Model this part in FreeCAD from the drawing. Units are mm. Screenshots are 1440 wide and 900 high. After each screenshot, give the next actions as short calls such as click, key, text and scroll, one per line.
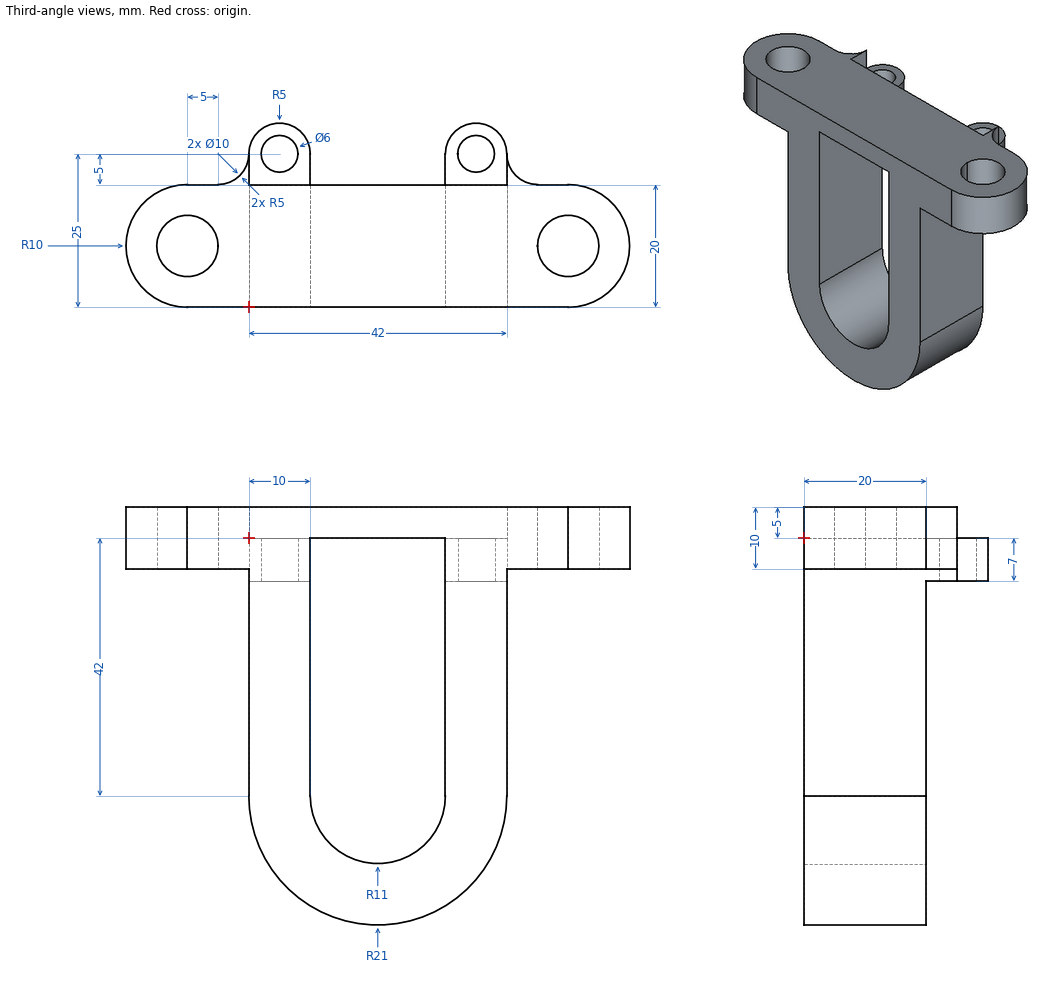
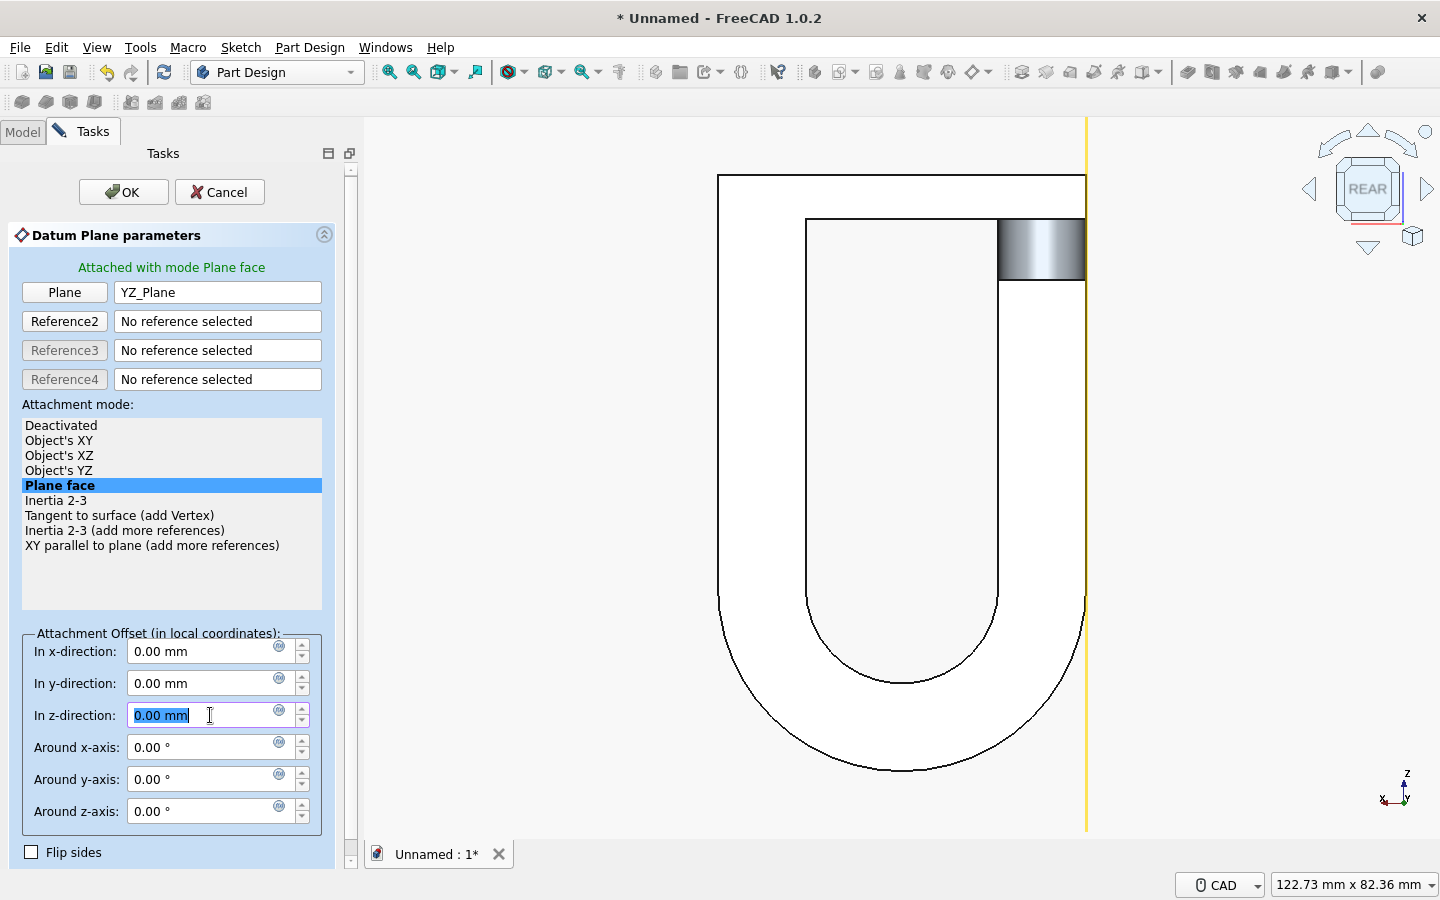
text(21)
key(Tab)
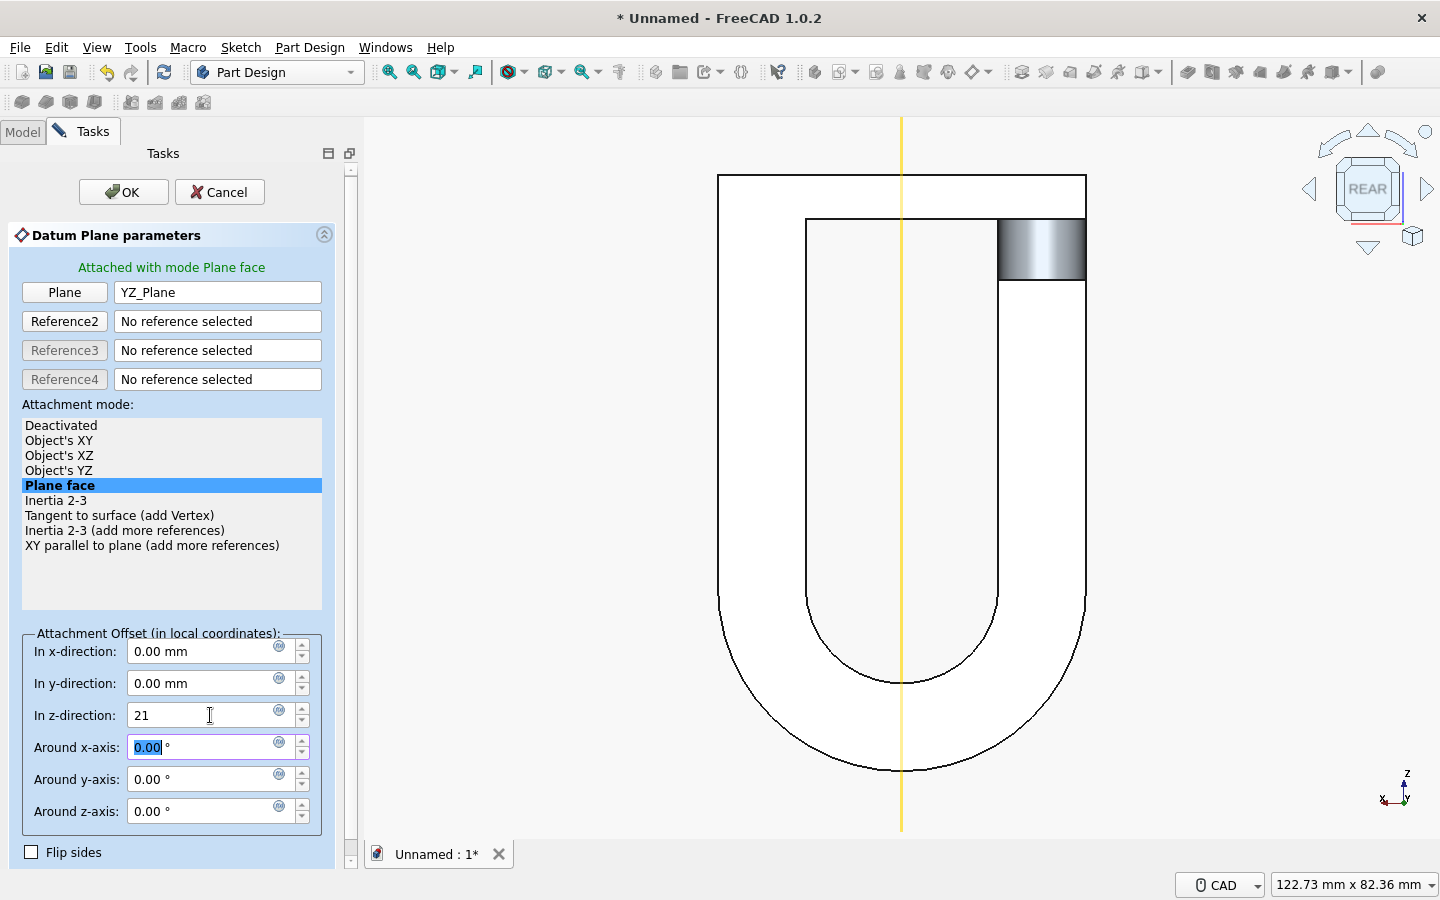
click(124, 192)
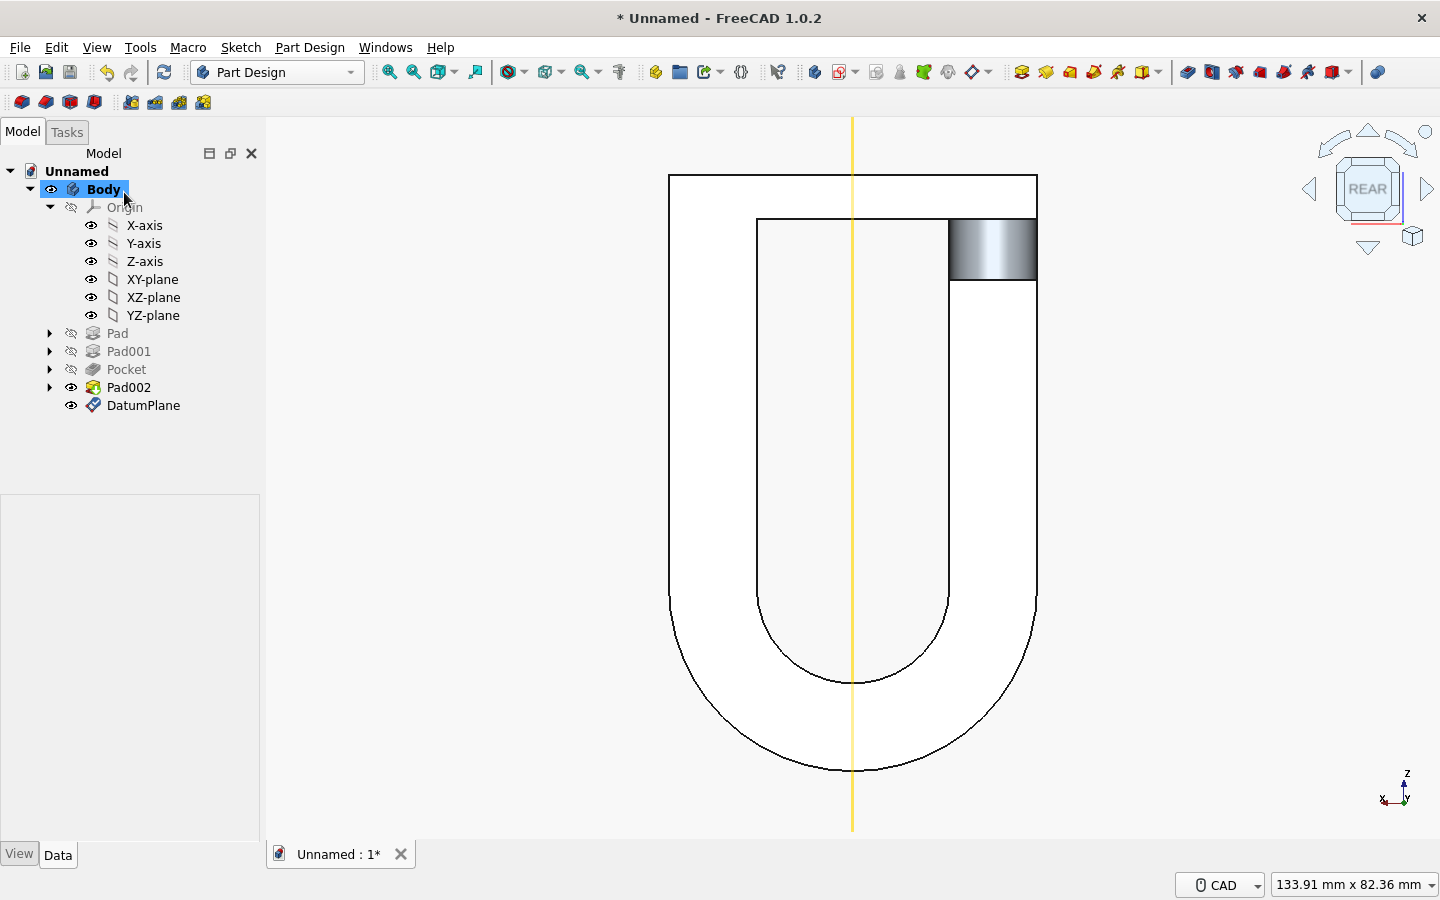
click(116, 387)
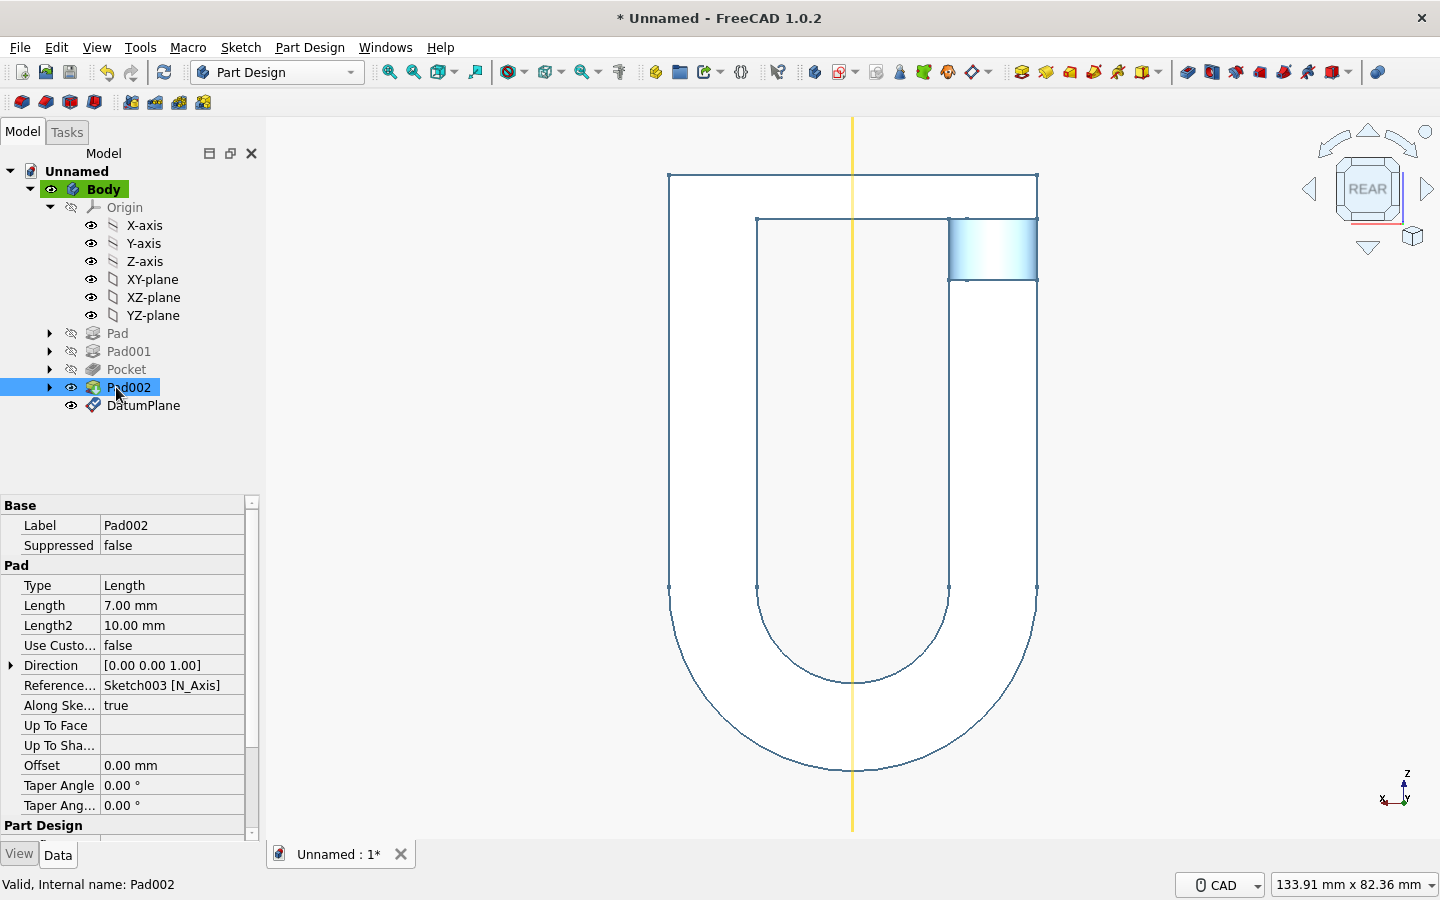
click(132, 102)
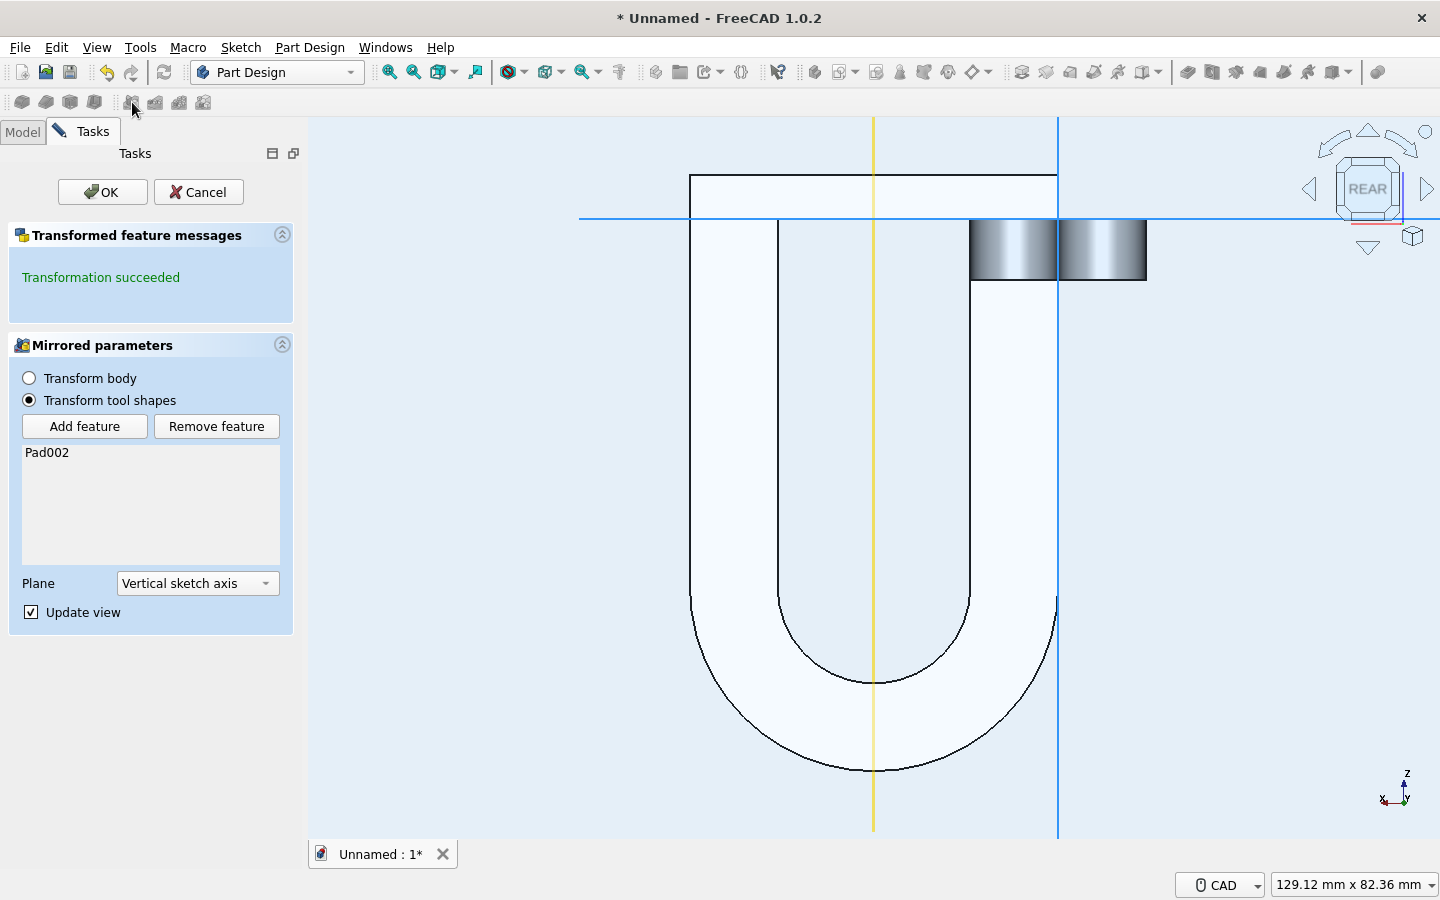
click(198, 584)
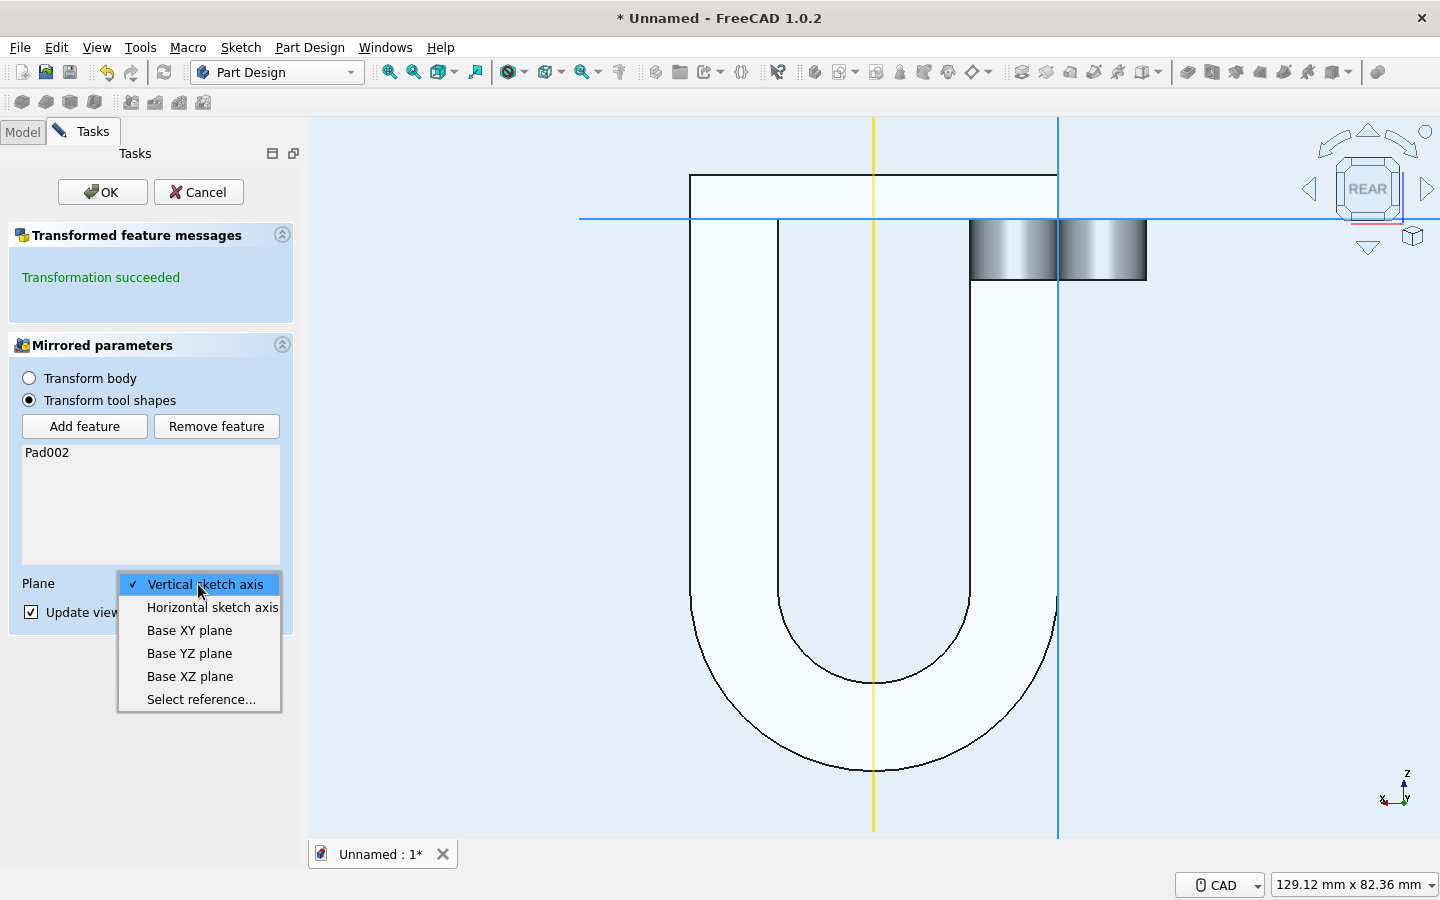
click(198, 700)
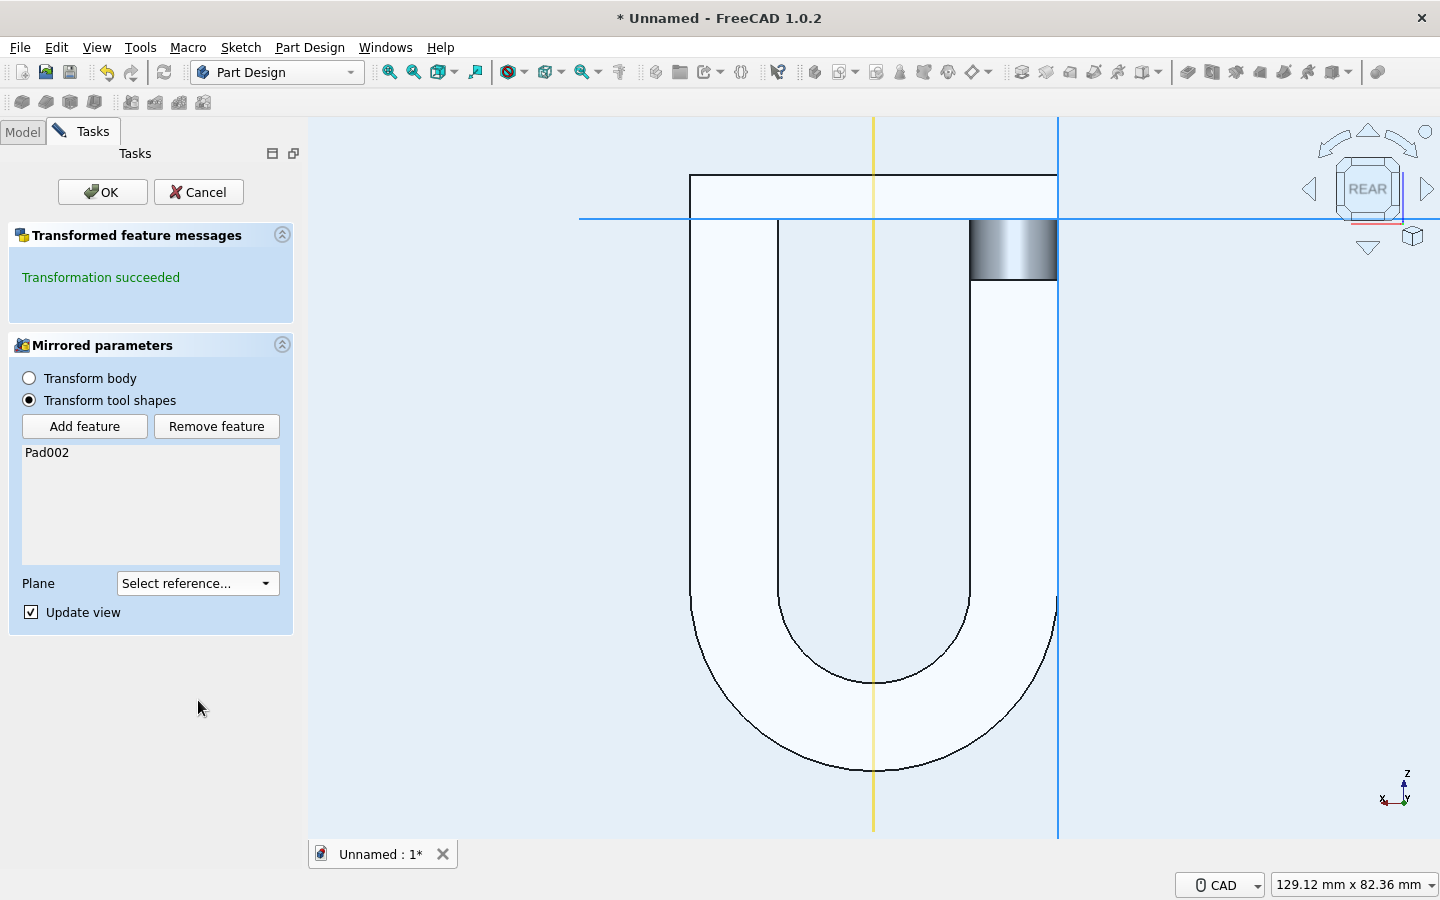
click(23, 131)